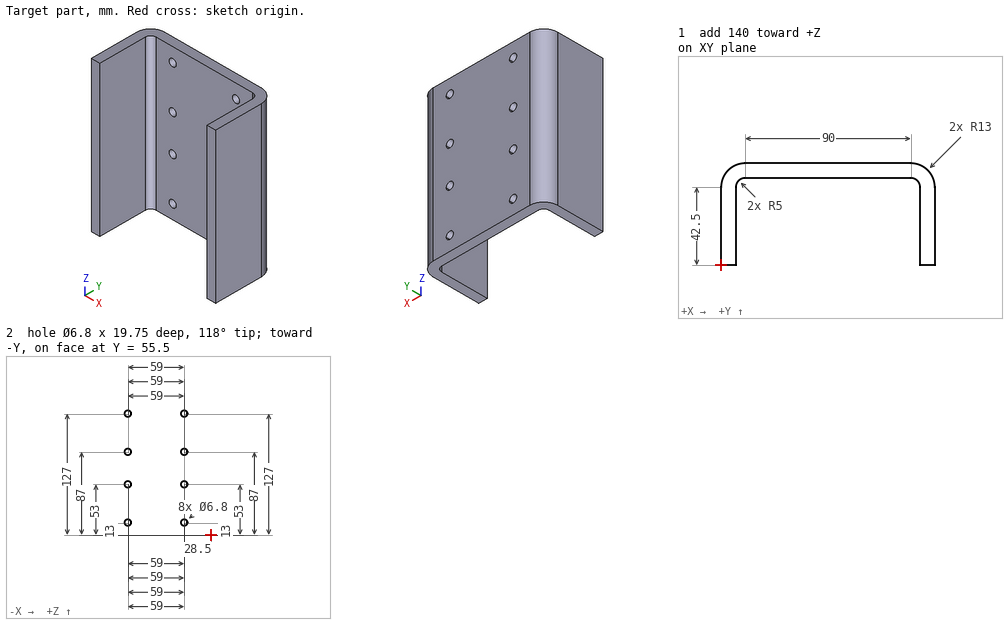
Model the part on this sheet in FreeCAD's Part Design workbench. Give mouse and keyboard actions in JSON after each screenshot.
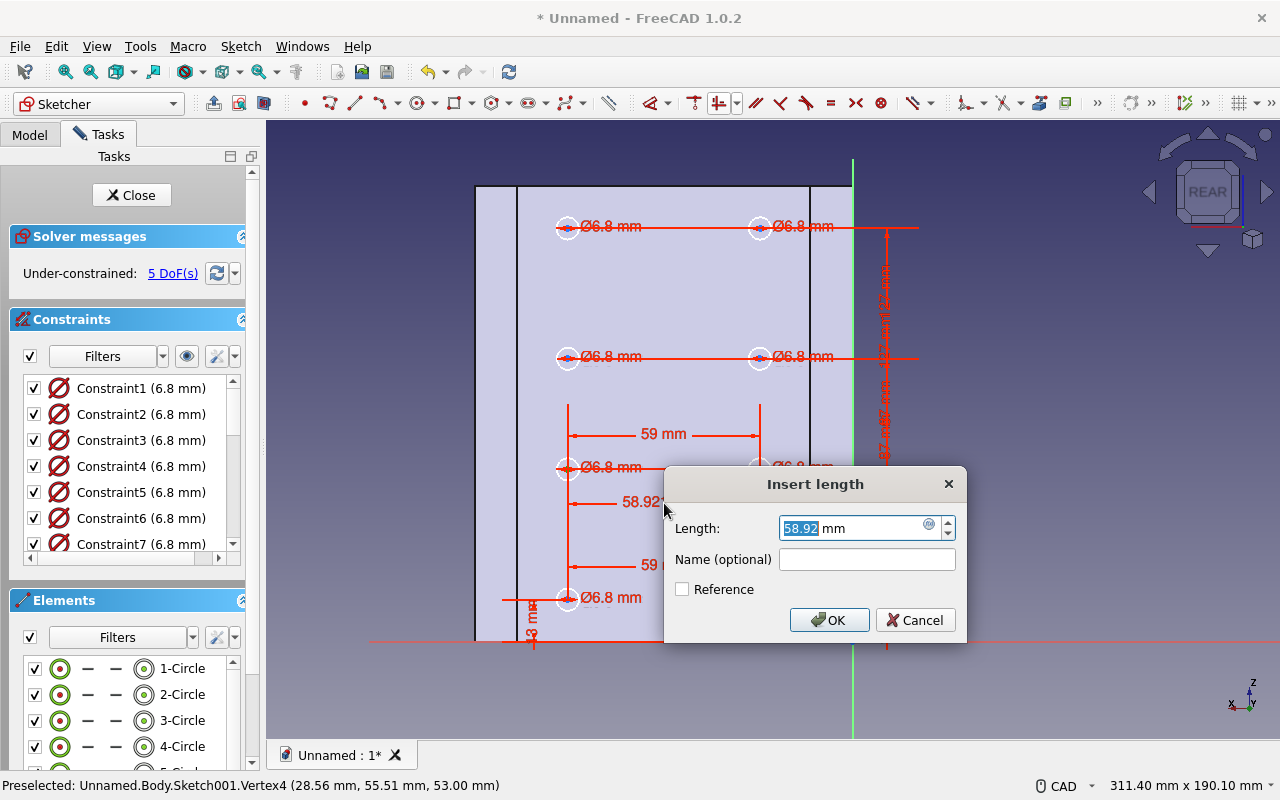
{"action": "type", "text": "59"}
{"action": "key", "text": "Return"}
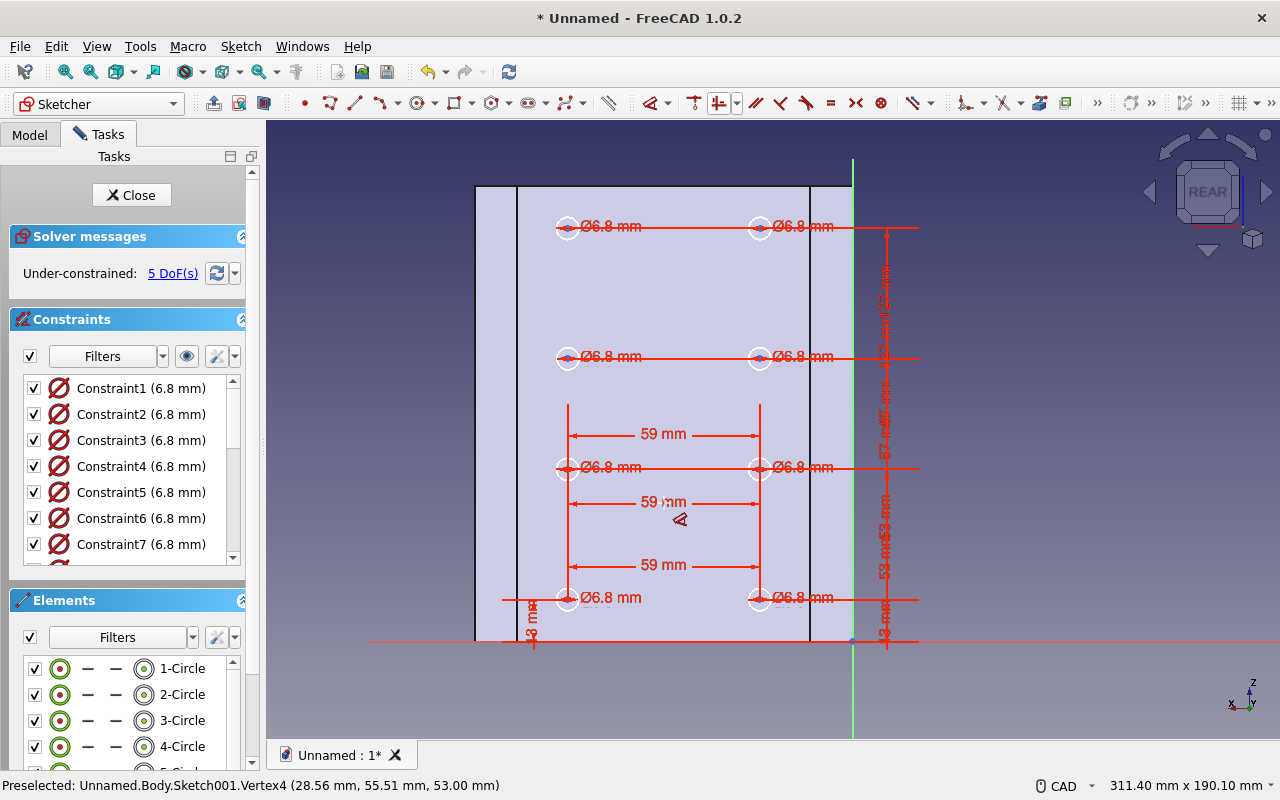
{"action": "left_click", "coordinate": [568, 469]}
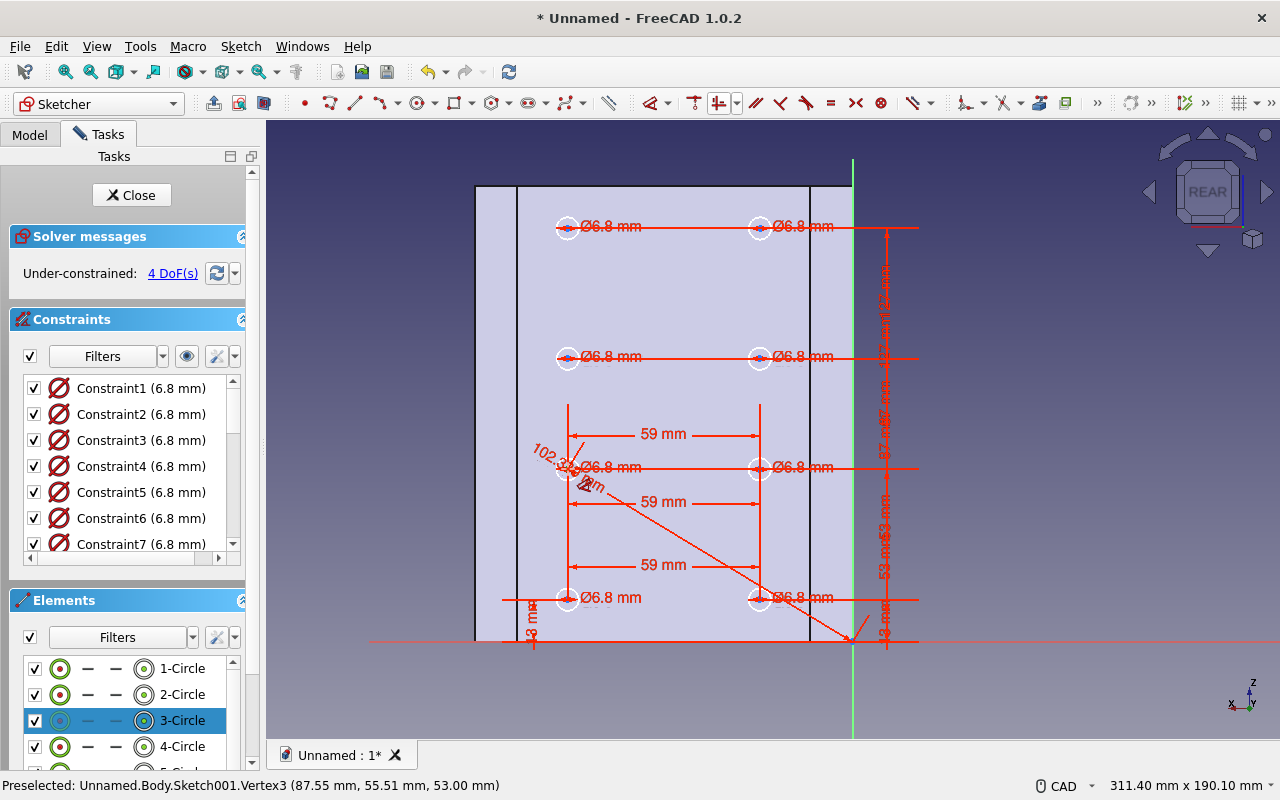
{"action": "left_click", "coordinate": [760, 359]}
{"action": "left_click", "coordinate": [664, 325]}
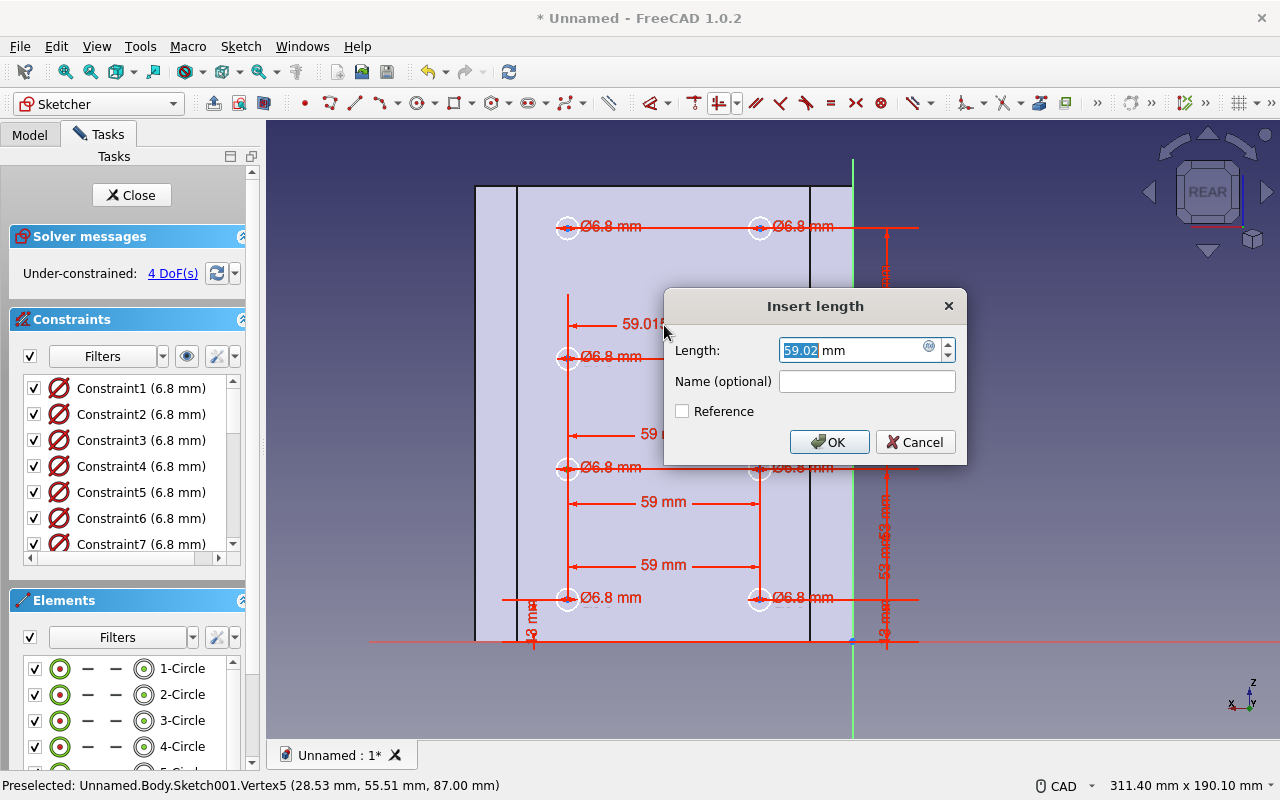
{"action": "type", "text": "59"}
{"action": "key", "text": "Return"}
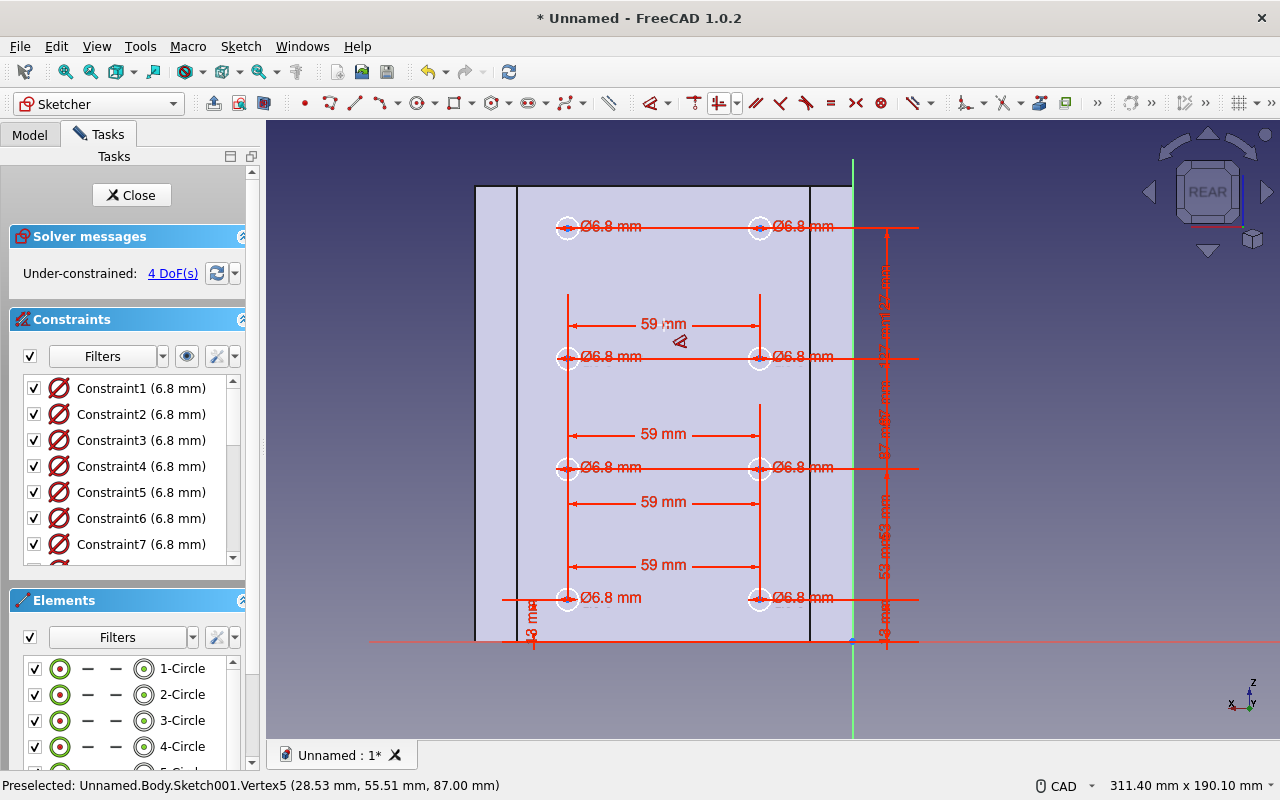
{"action": "left_click", "coordinate": [760, 359]}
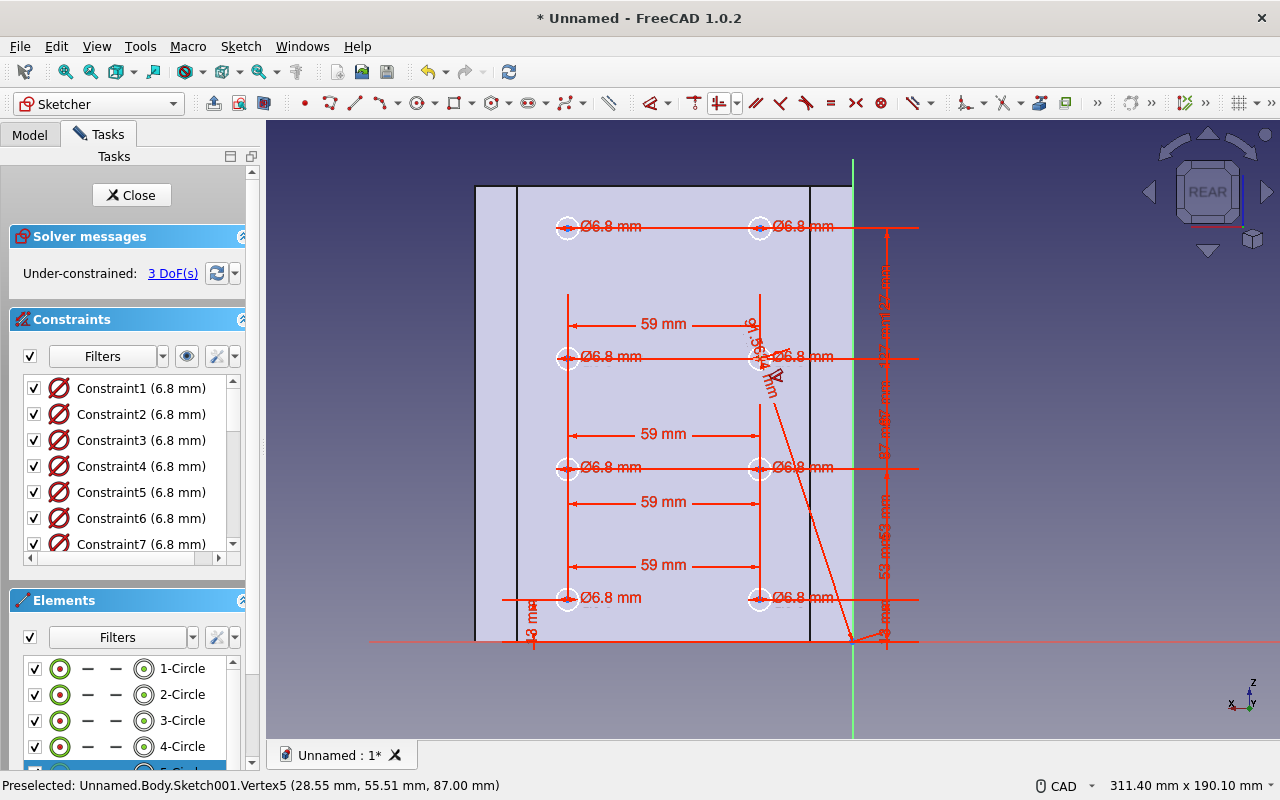
{"action": "left_click", "coordinate": [568, 359]}
{"action": "left_click", "coordinate": [664, 393]}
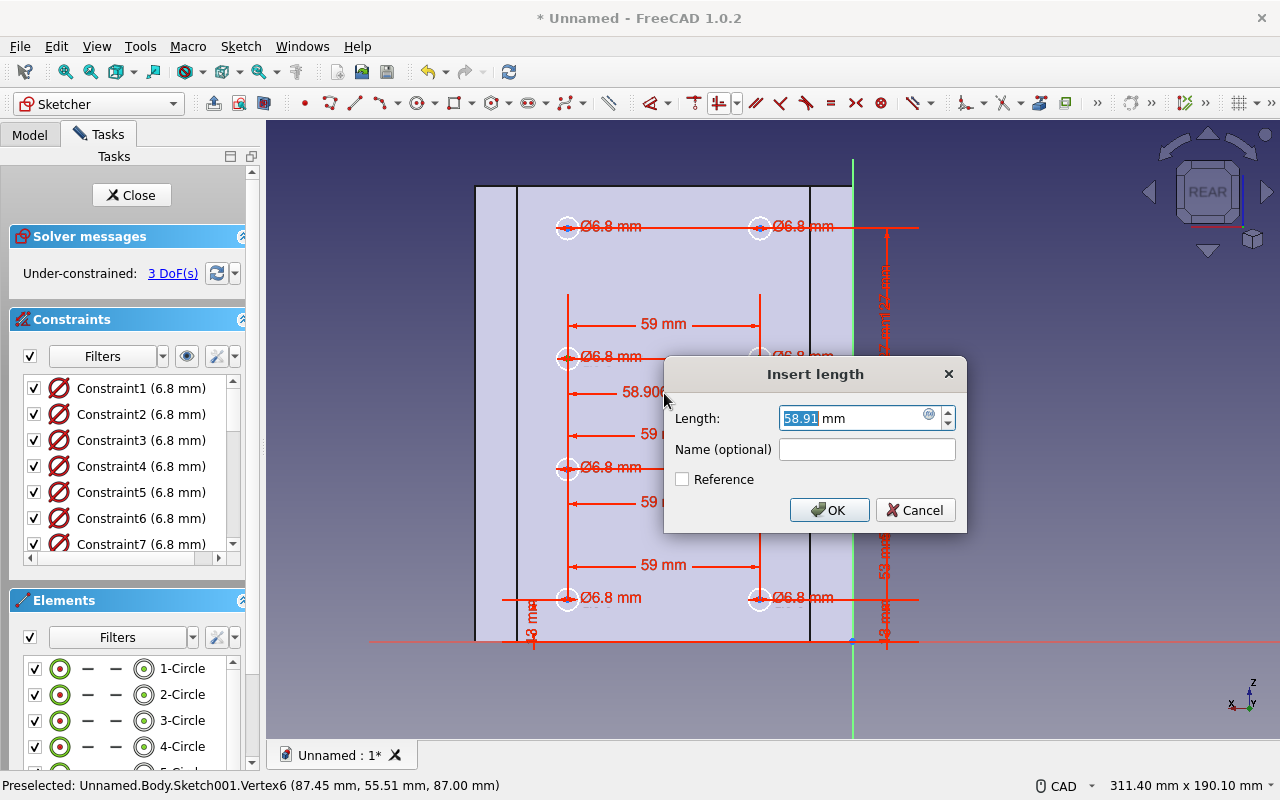
{"action": "type", "text": "59"}
{"action": "key", "text": "Return"}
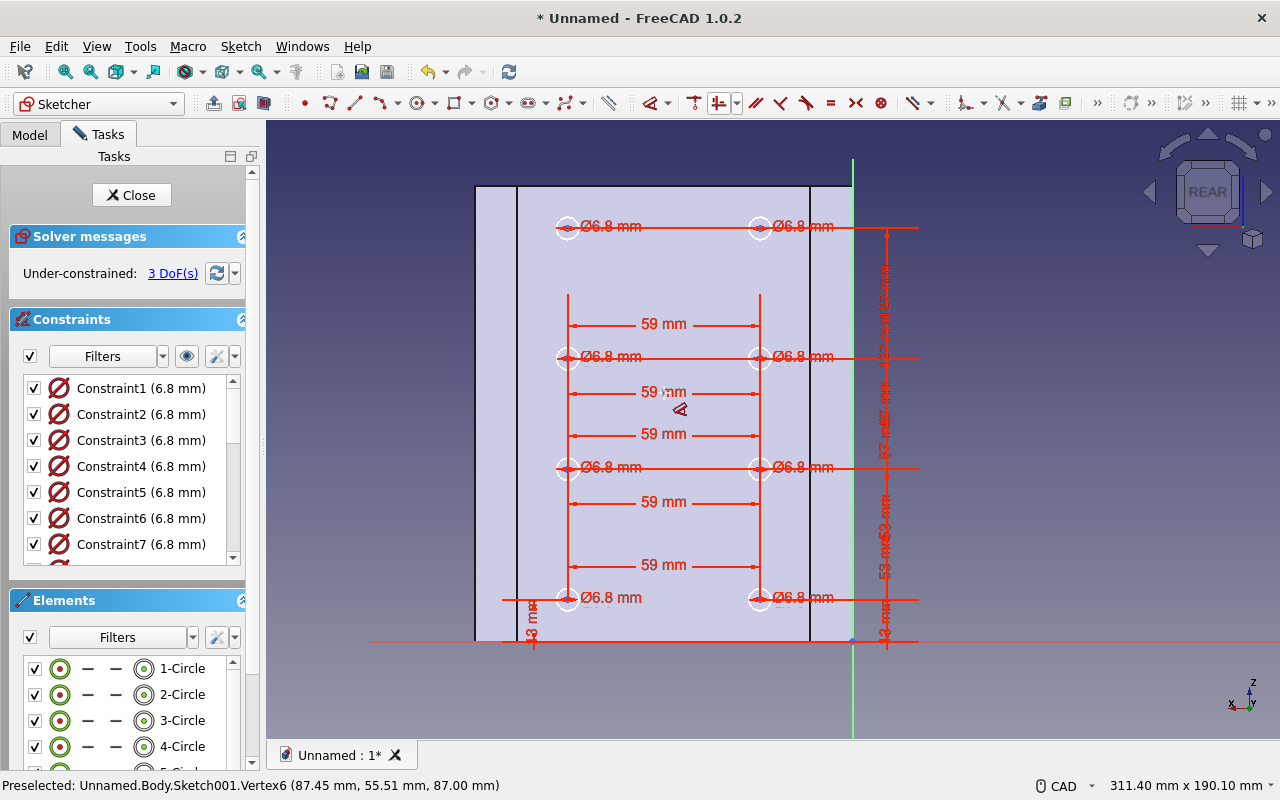
{"action": "left_click", "coordinate": [760, 359]}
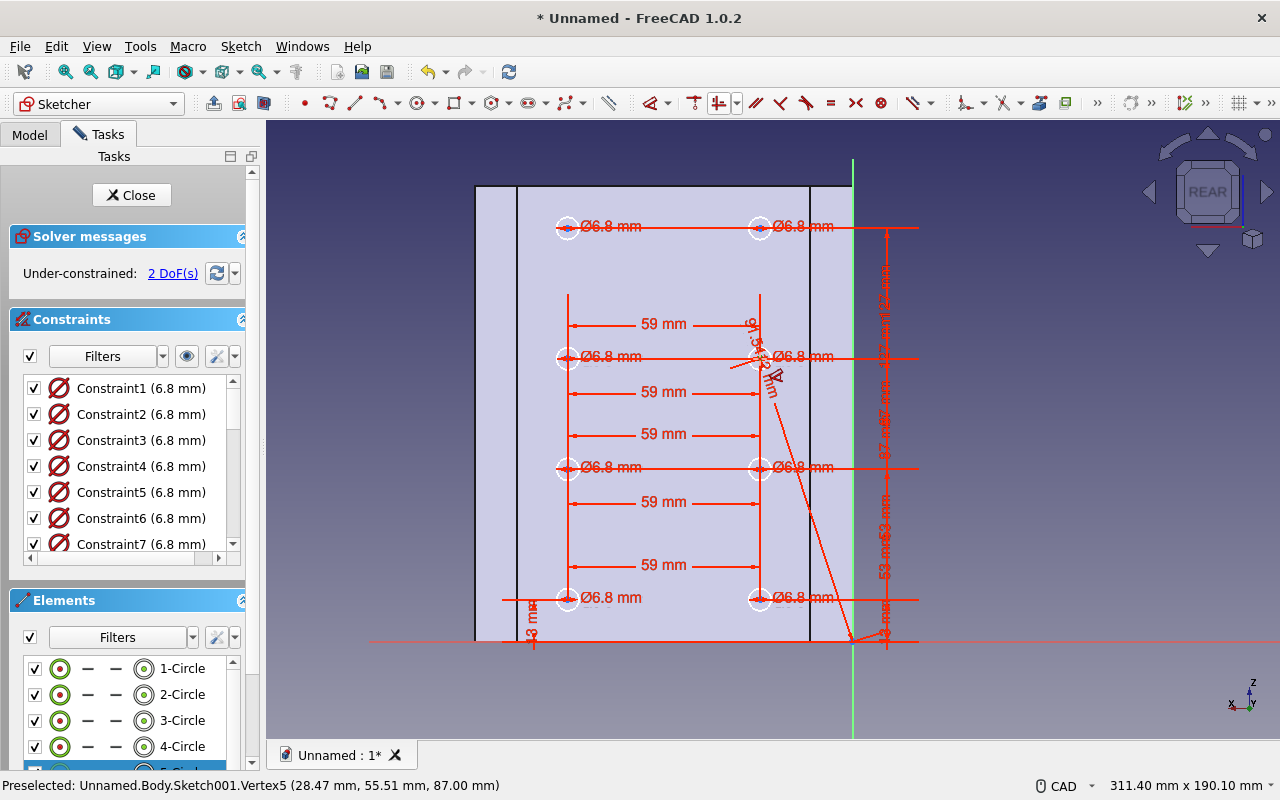
{"action": "left_click", "coordinate": [568, 228]}
{"action": "left_click", "coordinate": [664, 194]}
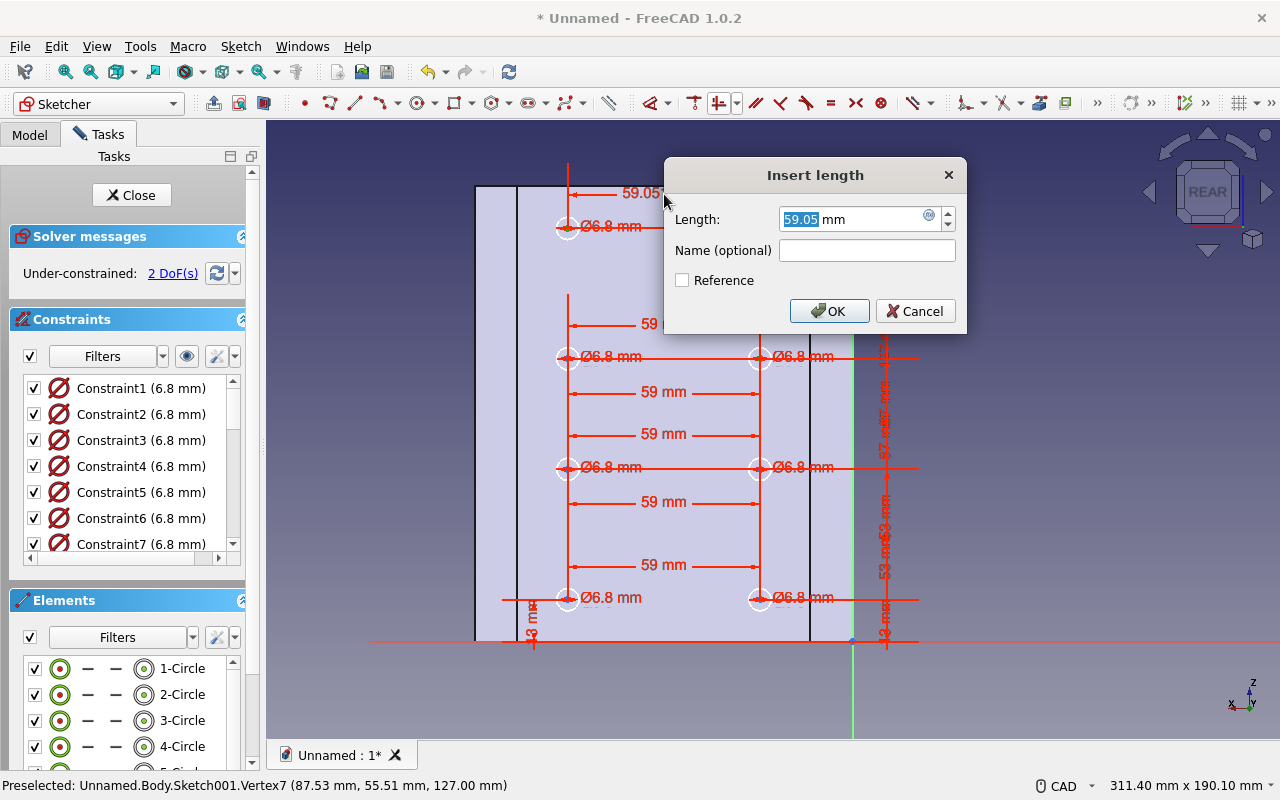
{"action": "type", "text": "59"}
{"action": "key", "text": "Return"}